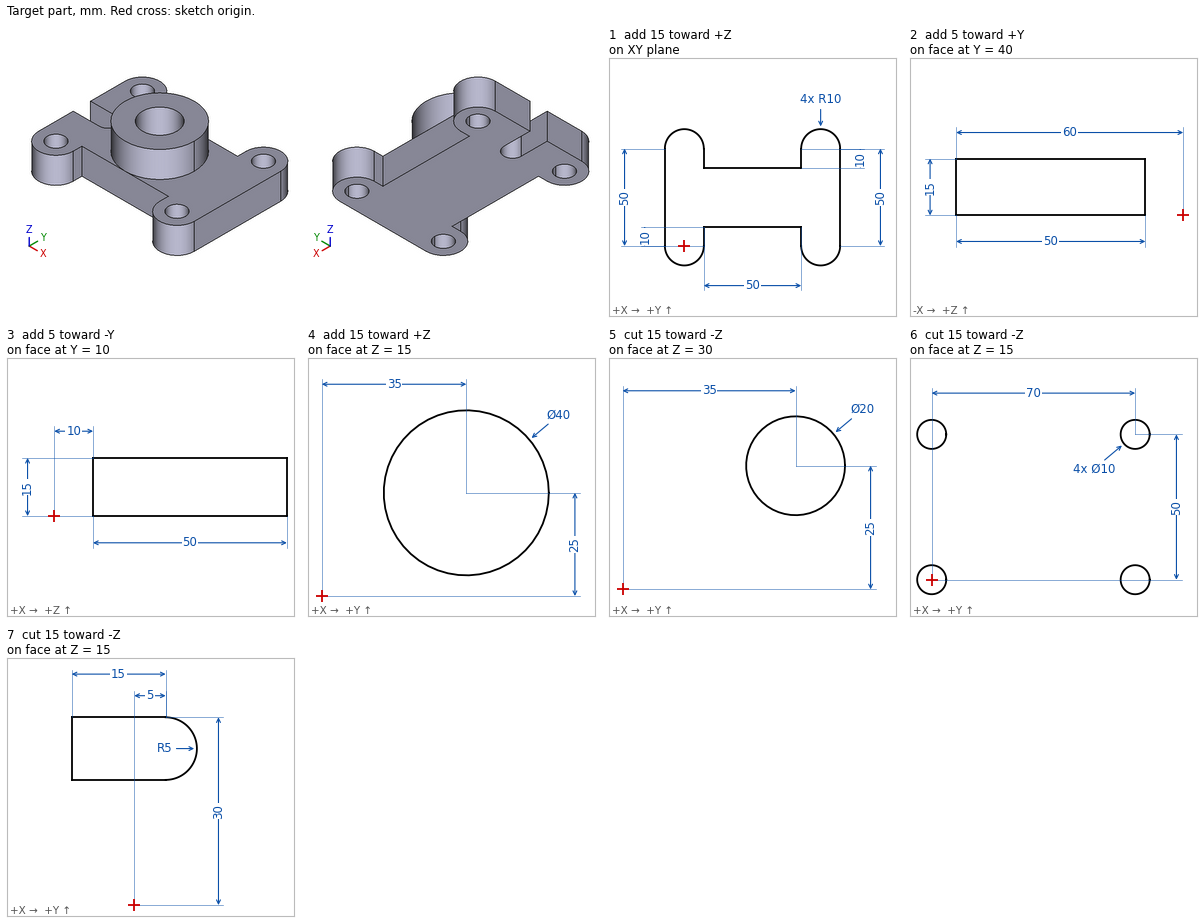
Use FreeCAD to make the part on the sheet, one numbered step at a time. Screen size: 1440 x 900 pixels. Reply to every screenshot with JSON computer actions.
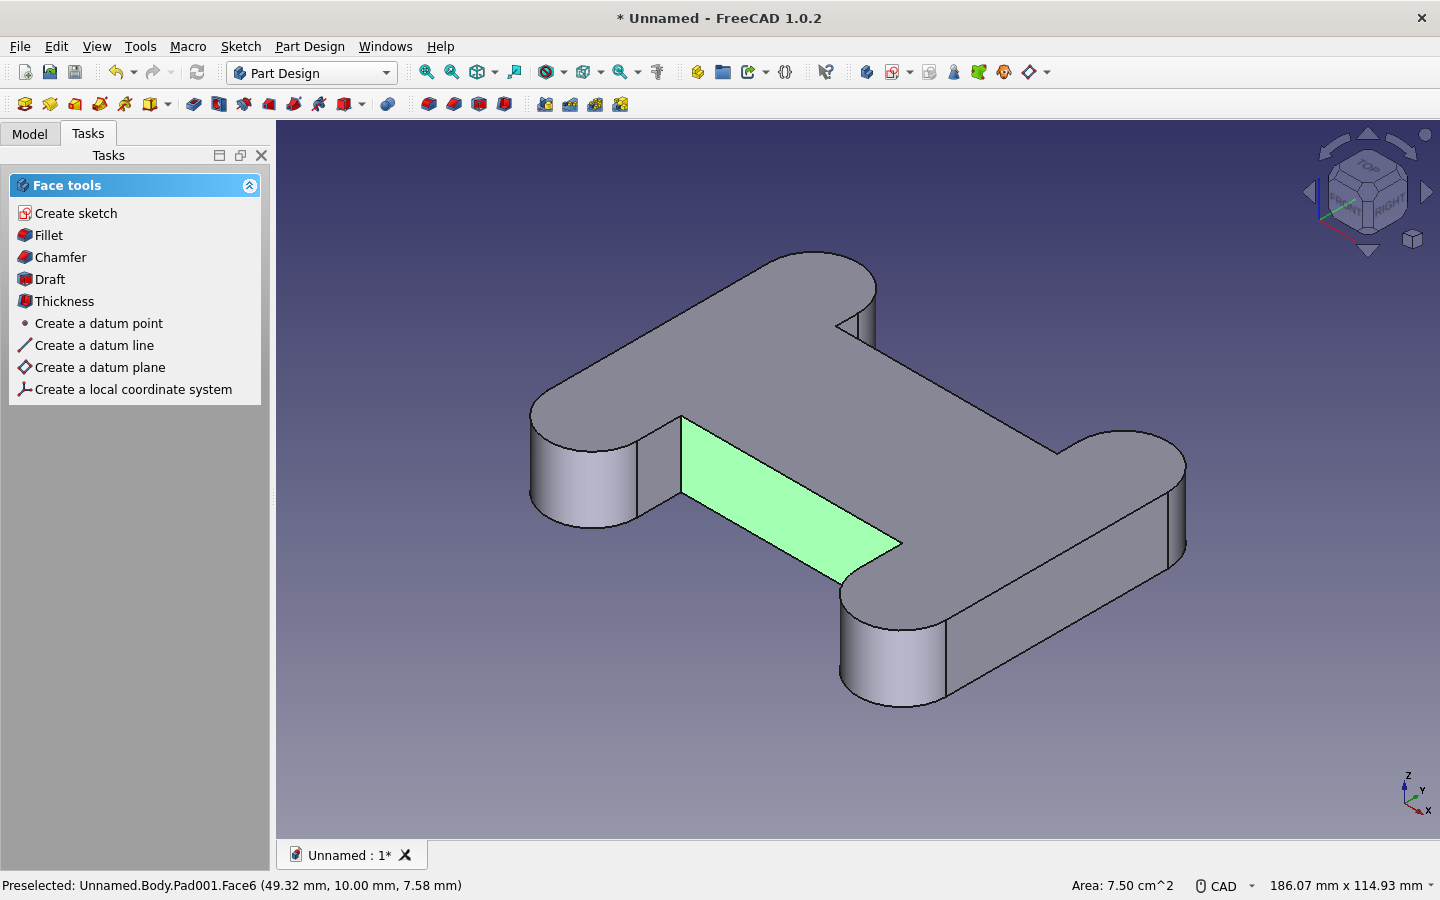
{"action": "left_click", "coordinate": [892, 72]}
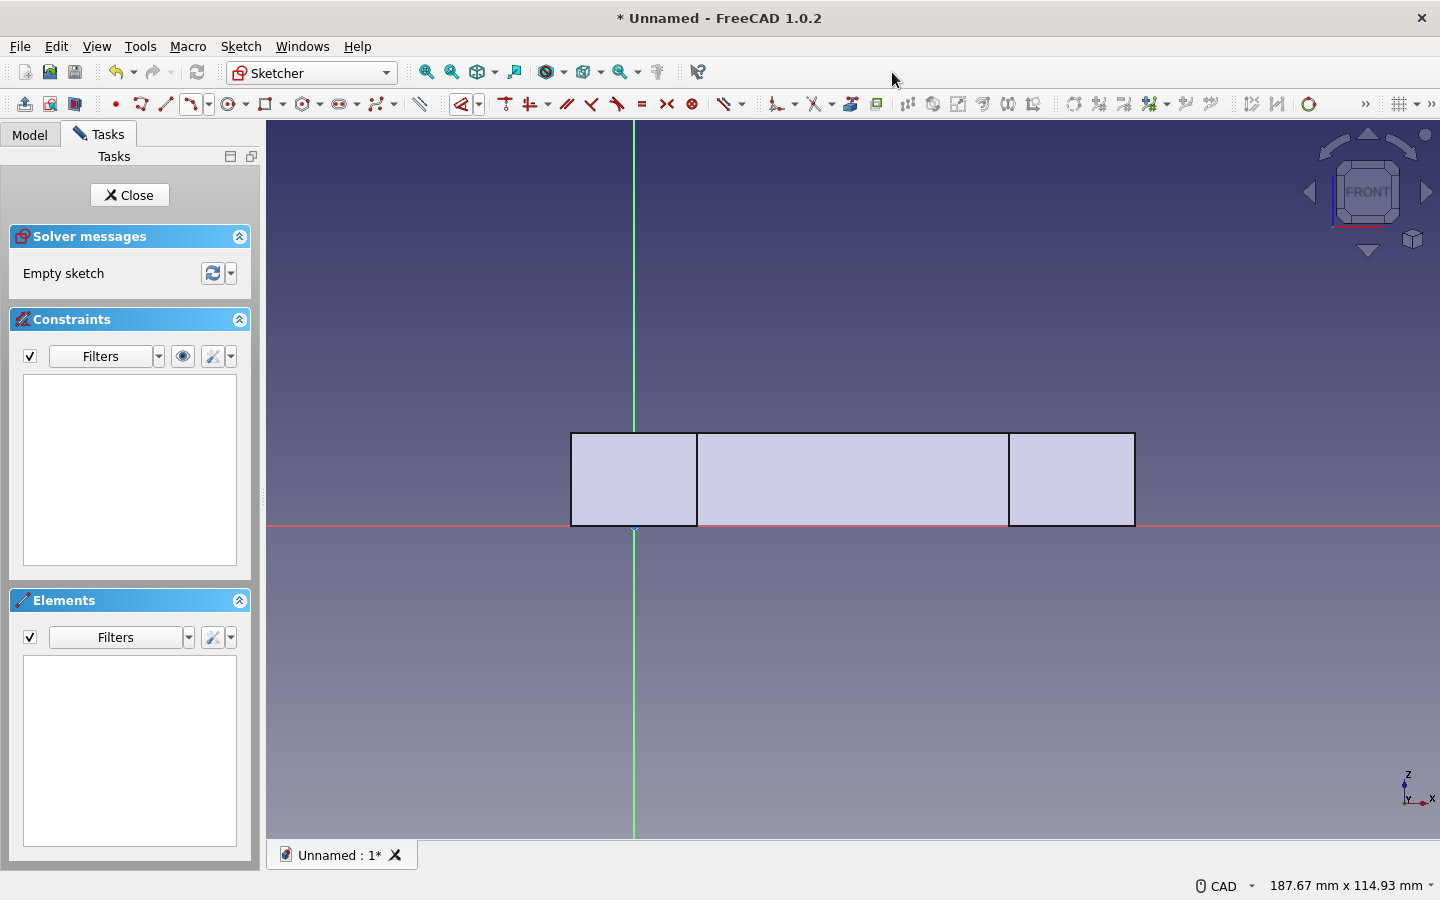
{"action": "scroll", "coordinate": [867, 480], "scroll_direction": "up", "scroll_amount": 3}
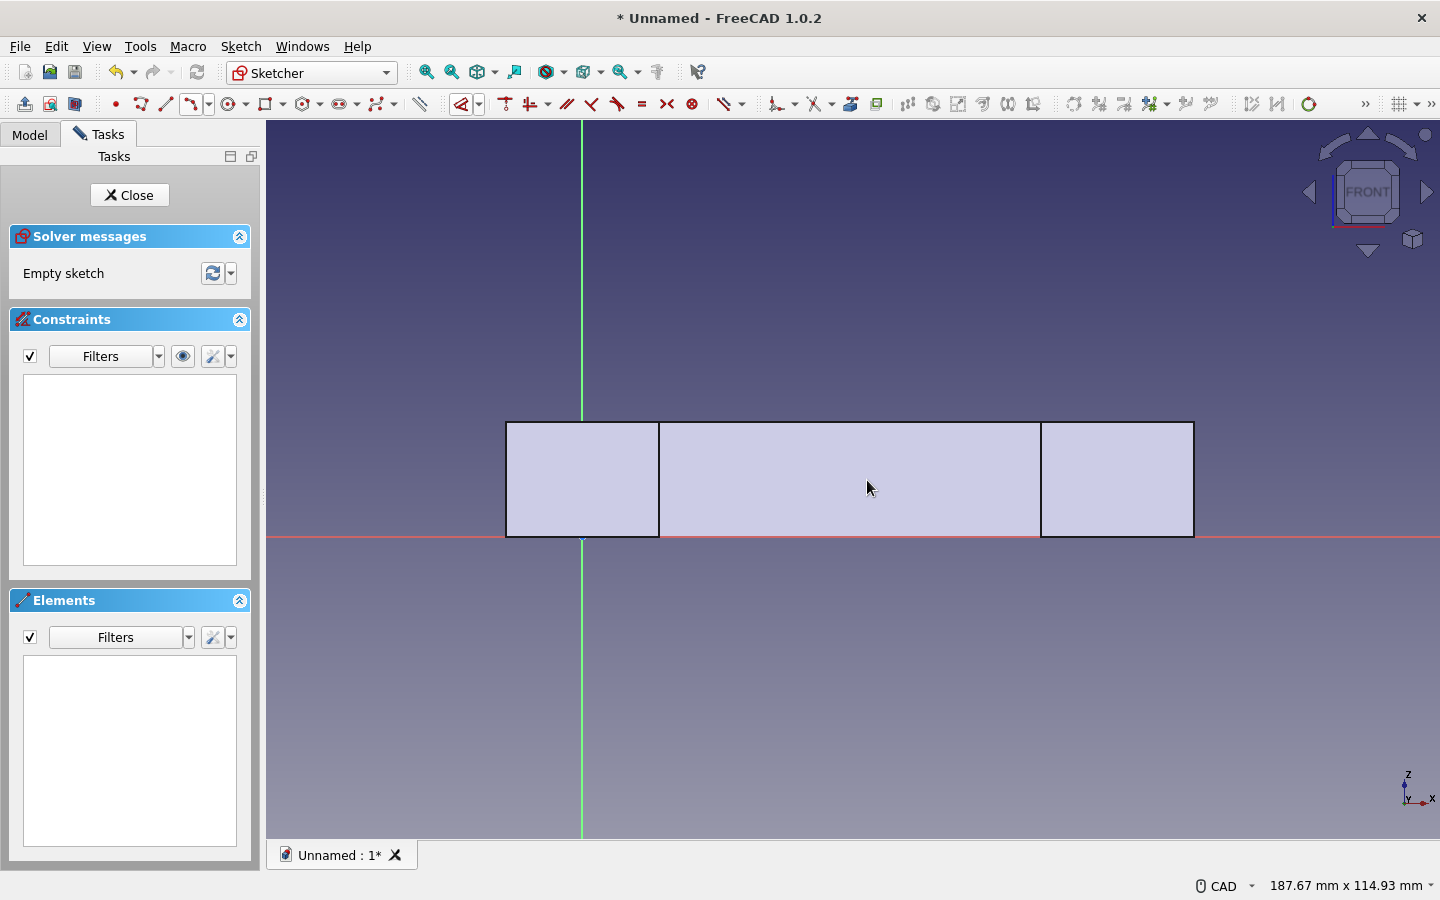
{"action": "key", "text": "g r"}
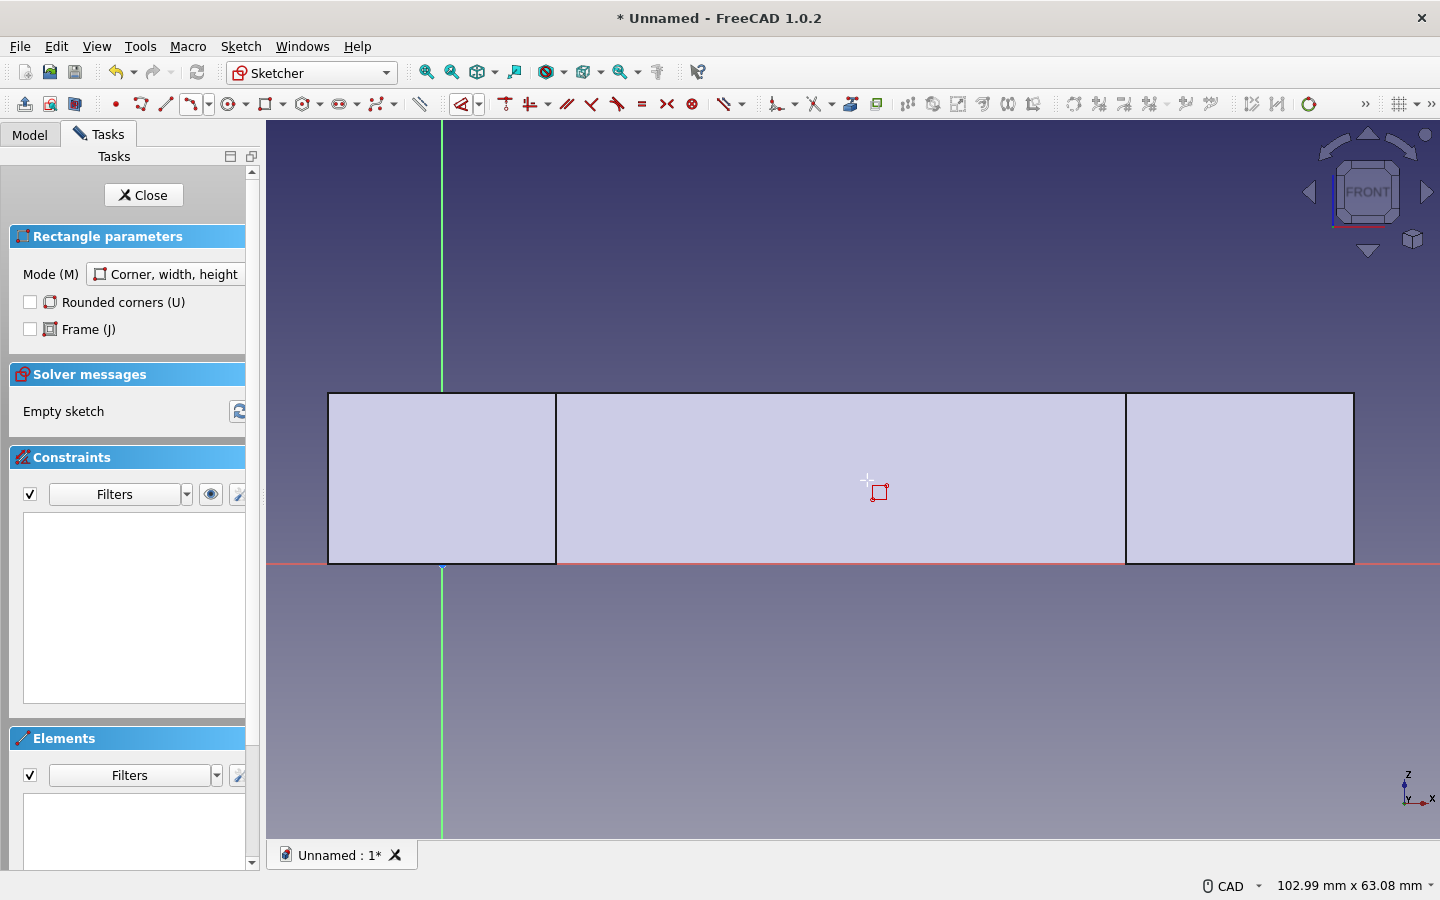
{"action": "left_click", "coordinate": [556, 393]}
{"action": "left_click", "coordinate": [1126, 564]}
{"action": "key", "text": "Escape"}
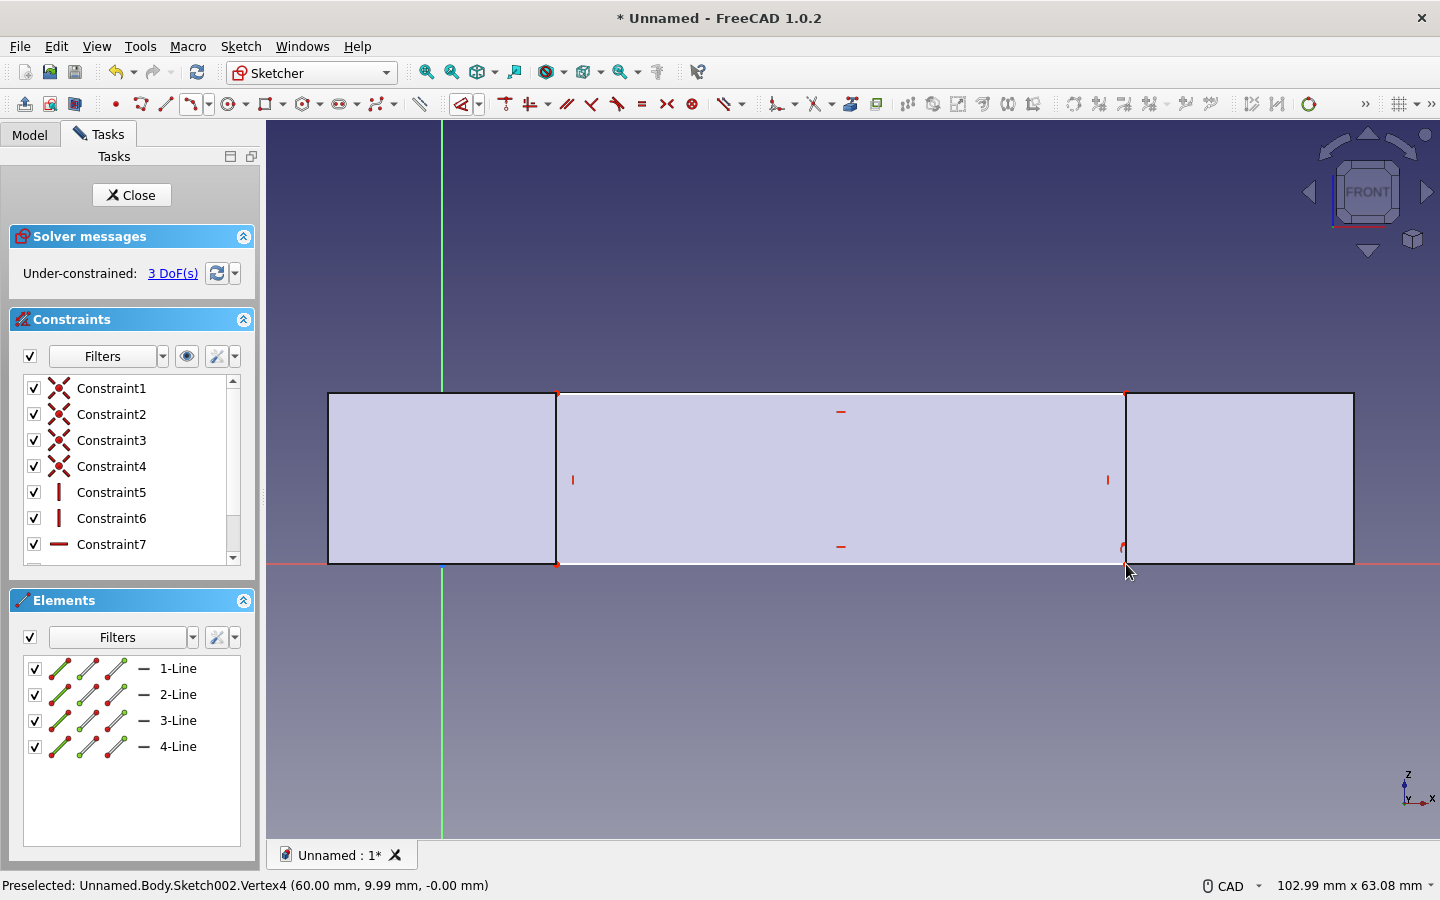
{"action": "left_click", "coordinate": [556, 445]}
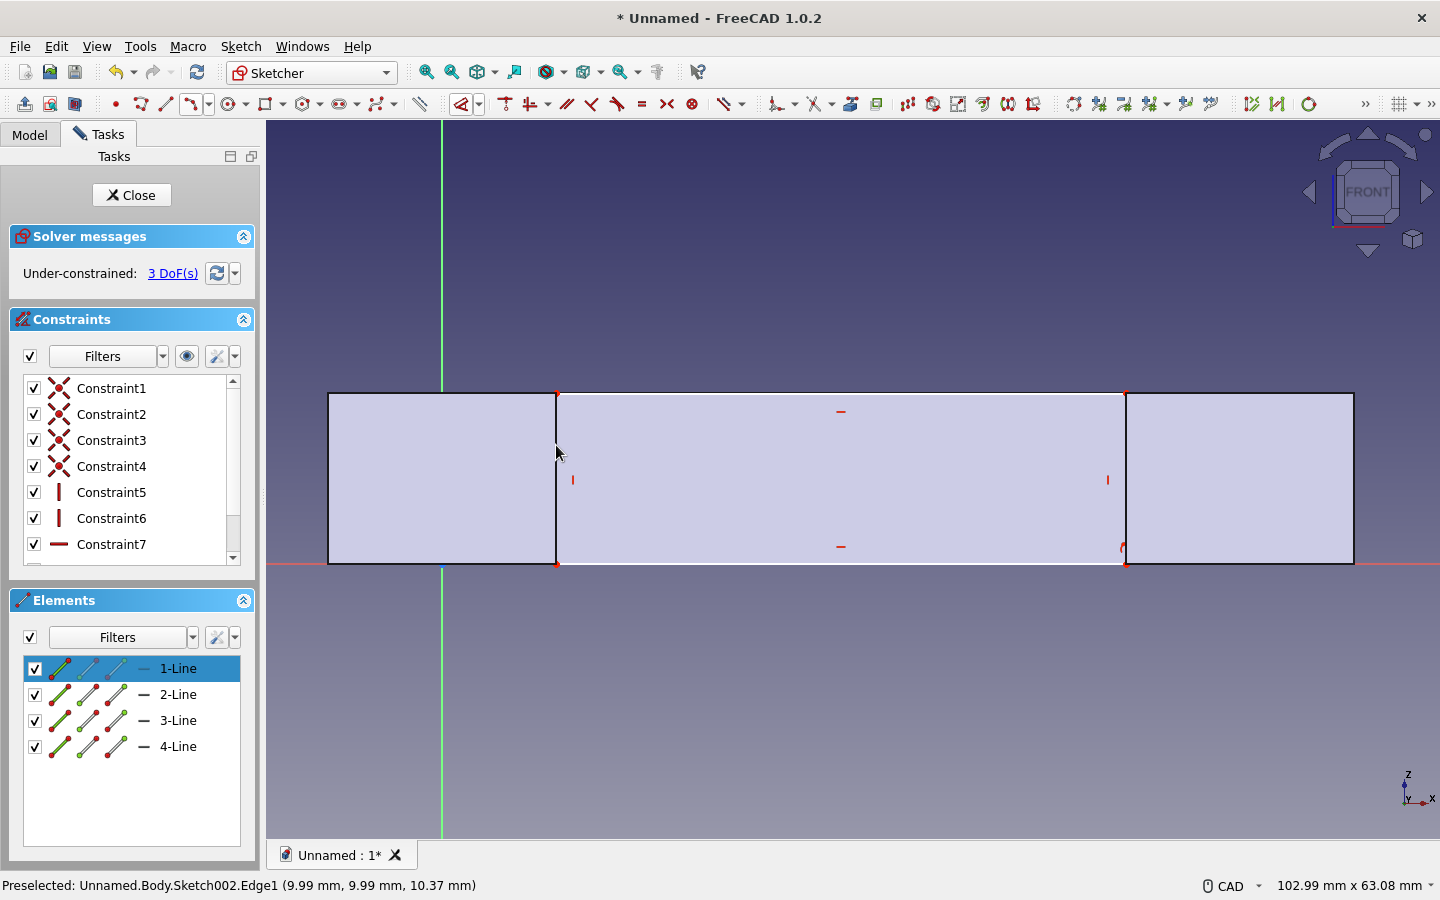
{"action": "left_click", "coordinate": [478, 104]}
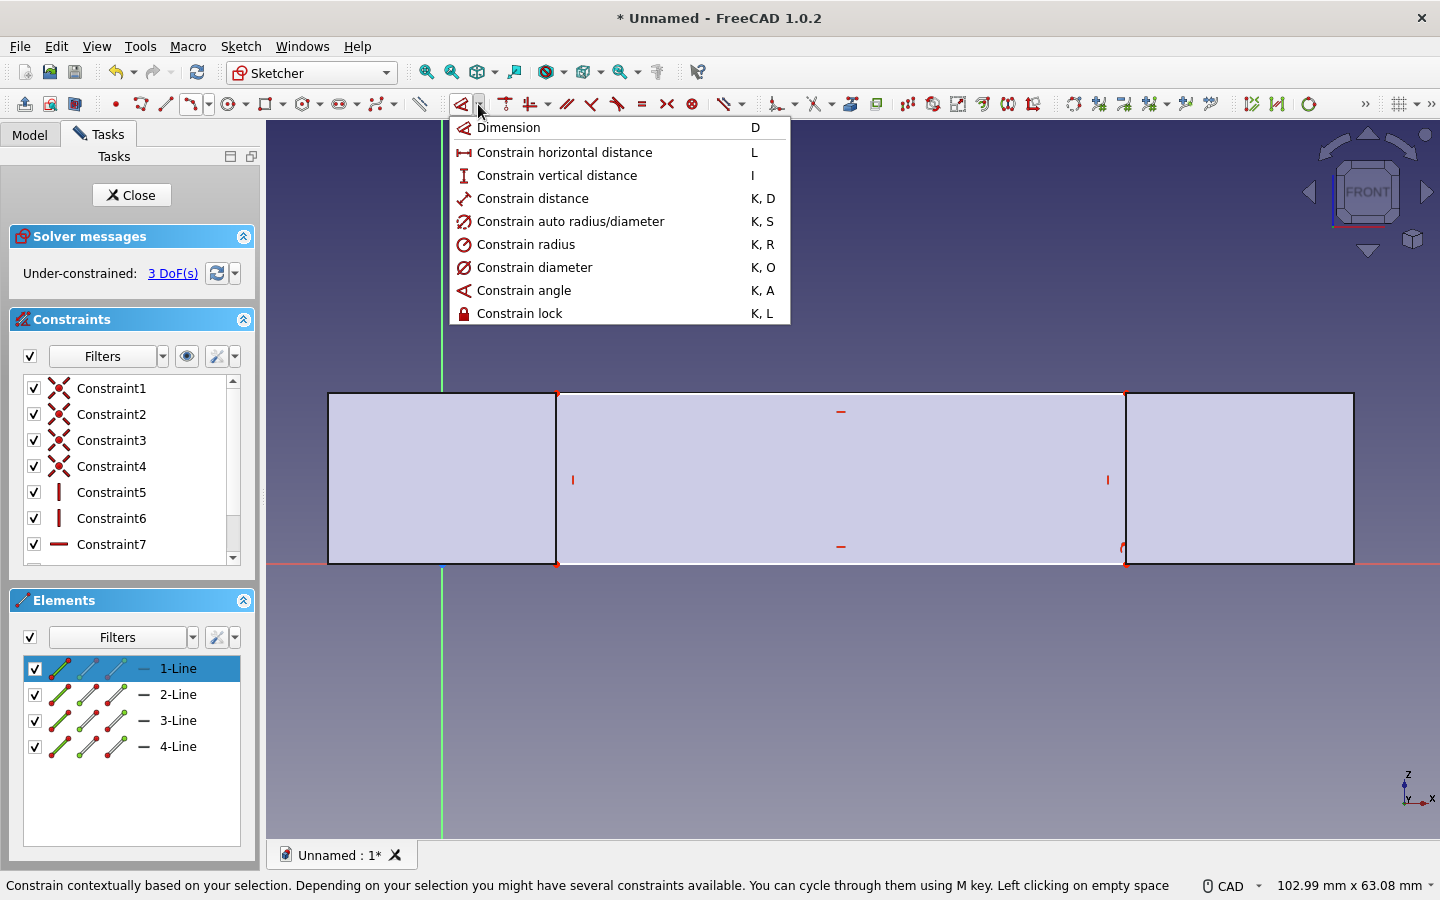
{"action": "left_click", "coordinate": [620, 176]}